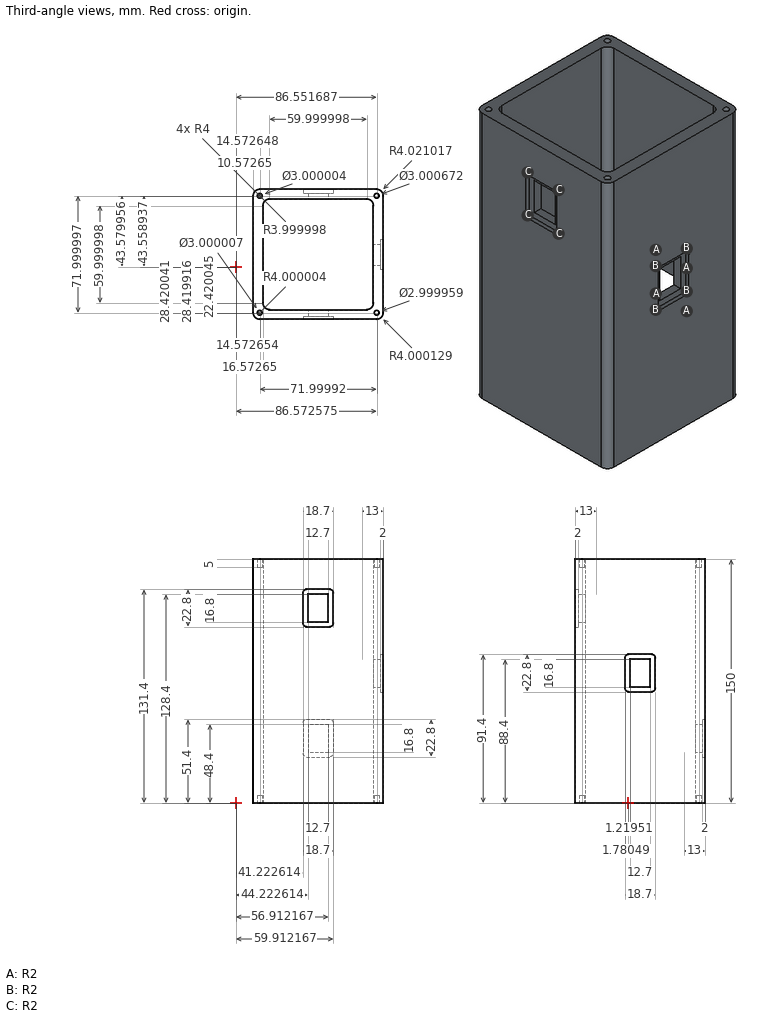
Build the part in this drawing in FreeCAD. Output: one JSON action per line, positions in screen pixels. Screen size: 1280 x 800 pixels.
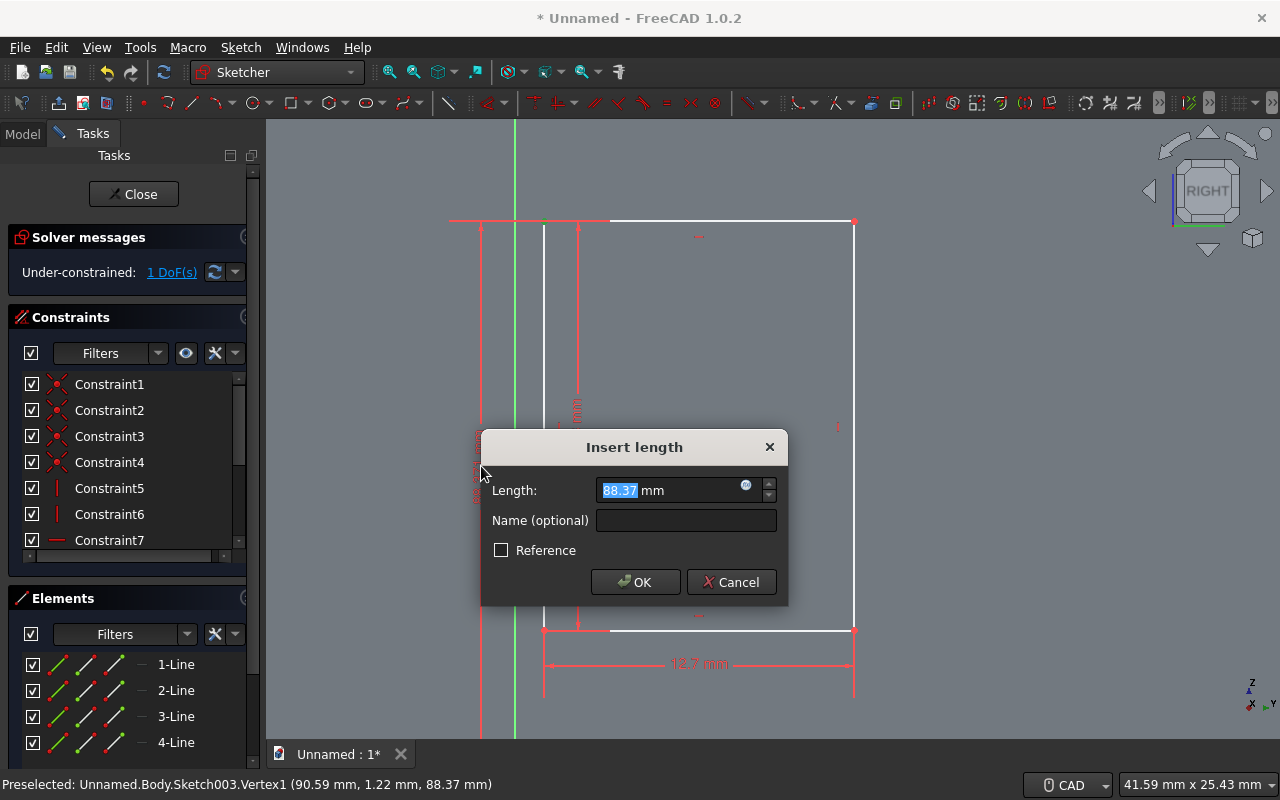
{"action": "type", "text": "88.4"}
{"action": "key", "text": "Return"}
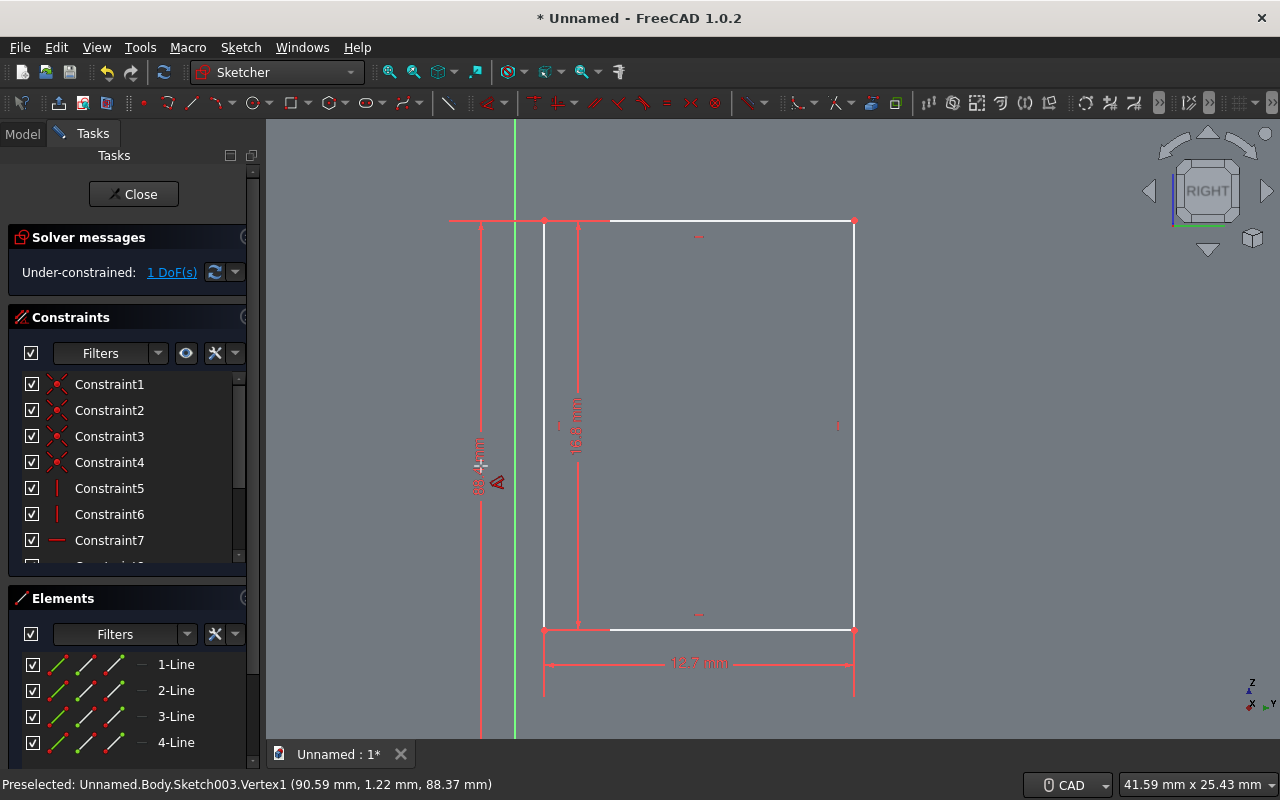
{"action": "scroll", "coordinate": [544, 221], "scroll_direction": "up", "scroll_amount": 2}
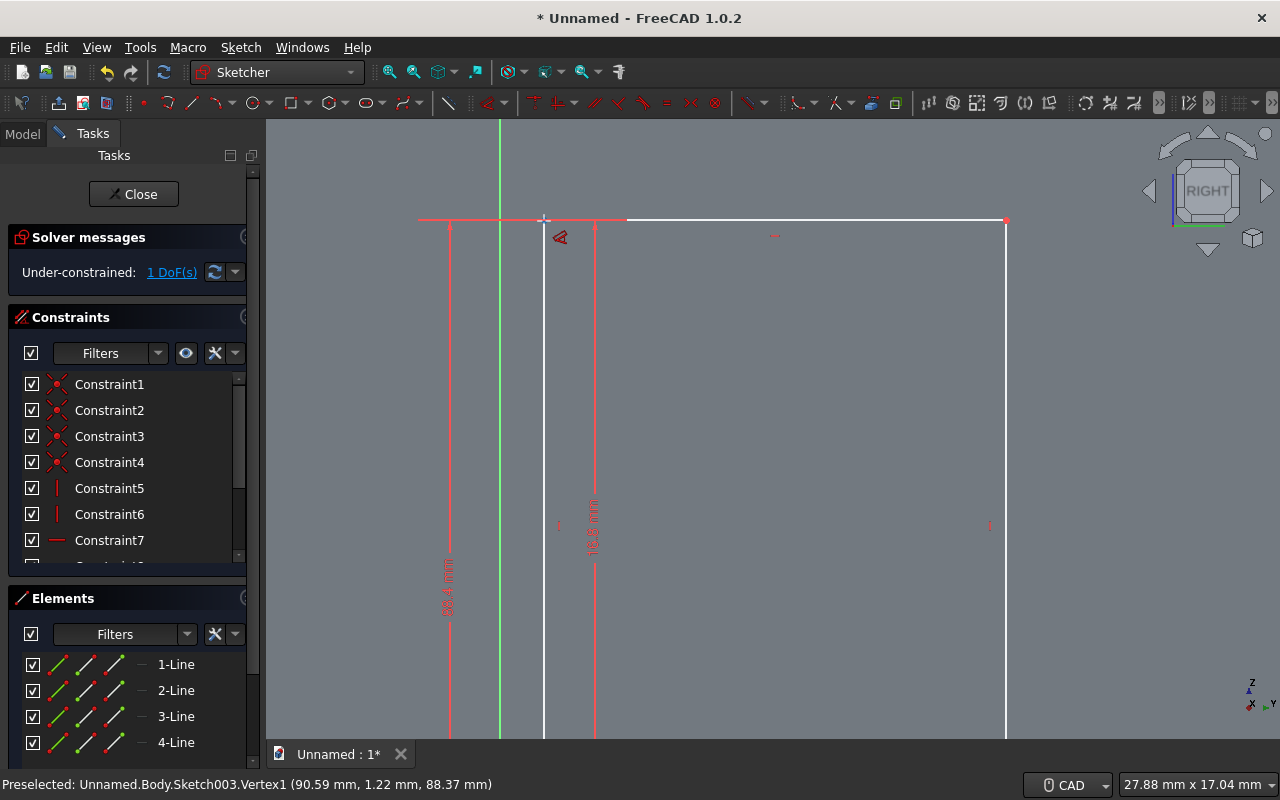
{"action": "left_click", "coordinate": [544, 220]}
{"action": "left_click", "coordinate": [522, 186]}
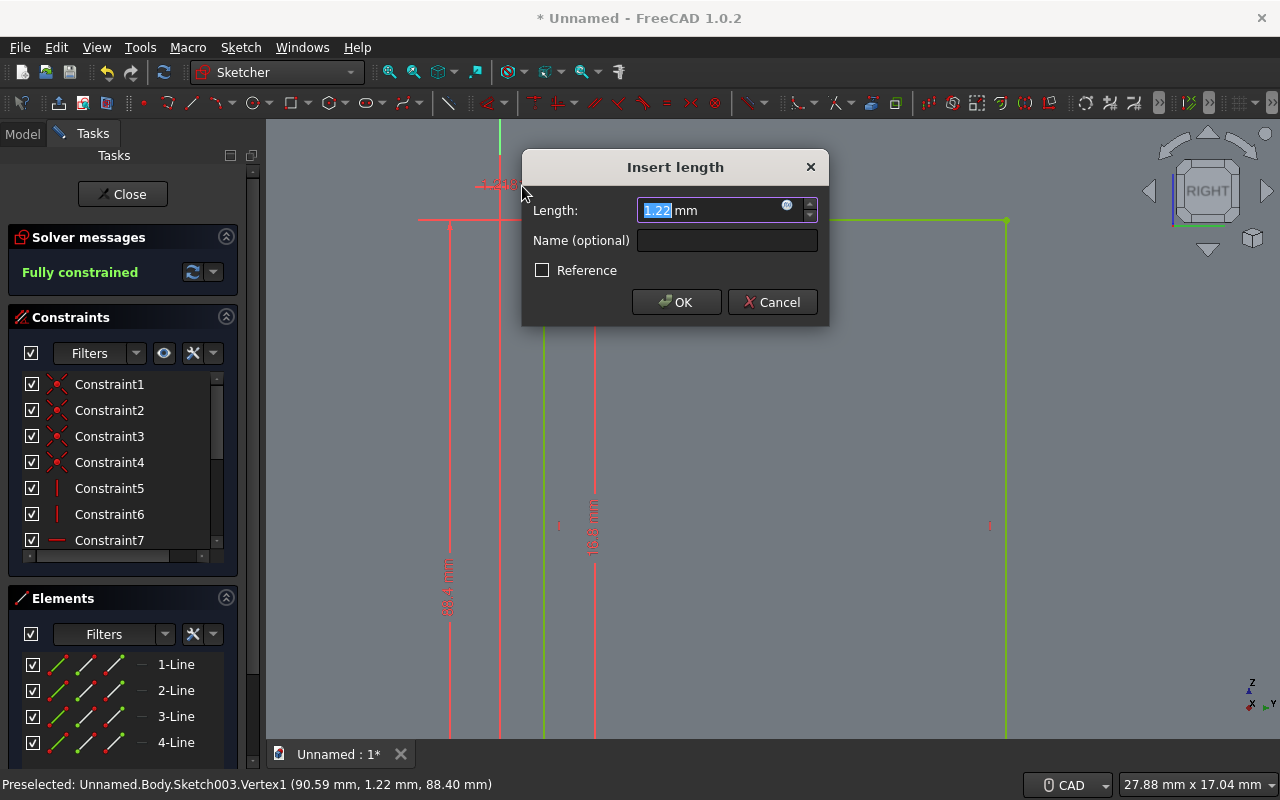
{"action": "type", "text": "1.21951"}
{"action": "key", "text": "Return"}
{"action": "key", "text": "Escape"}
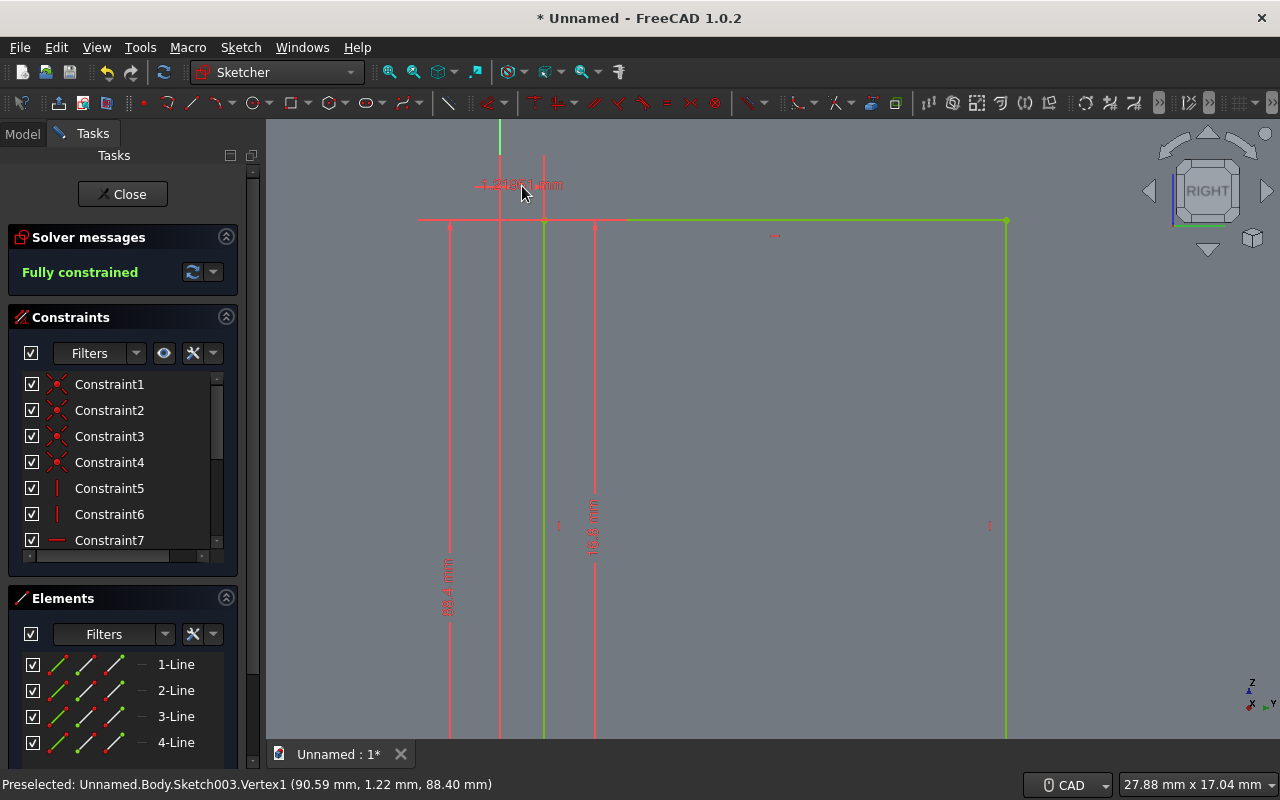
{"action": "left_click", "coordinate": [123, 194]}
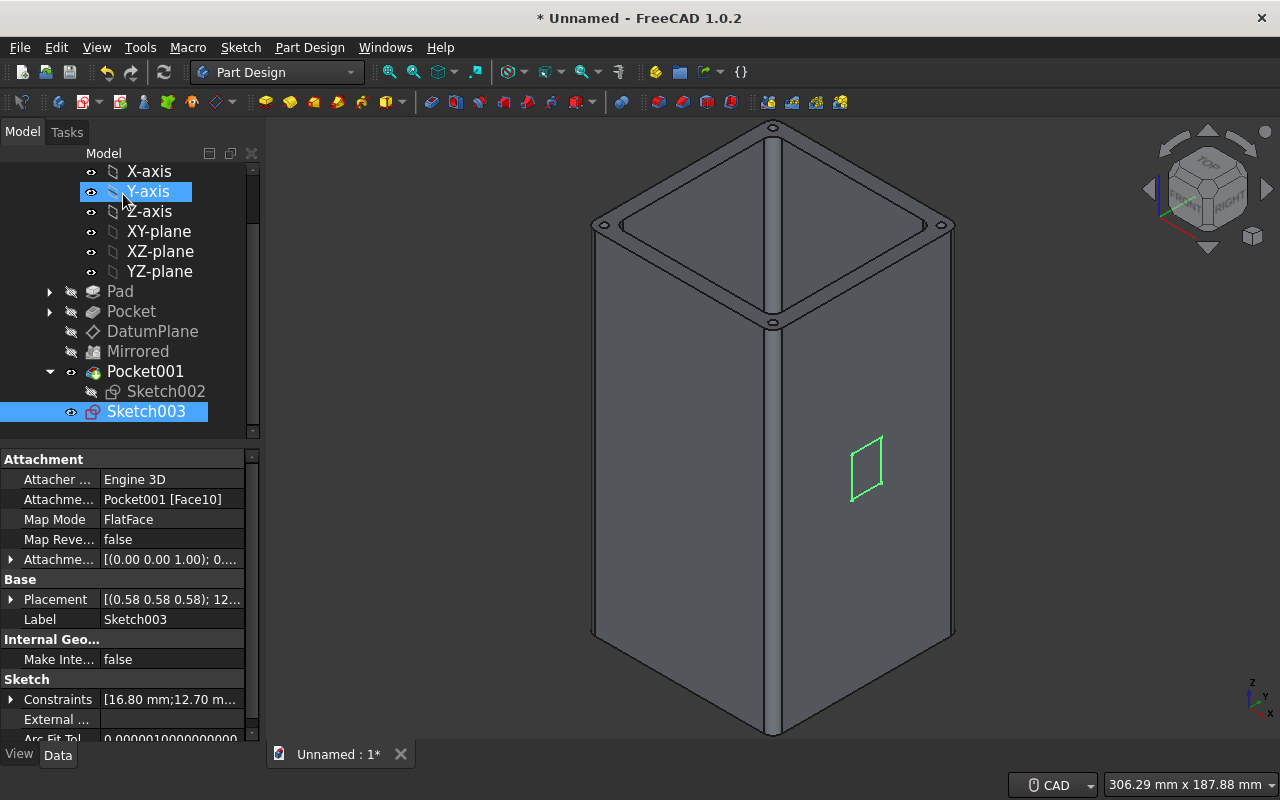
{"action": "left_click", "coordinate": [432, 102]}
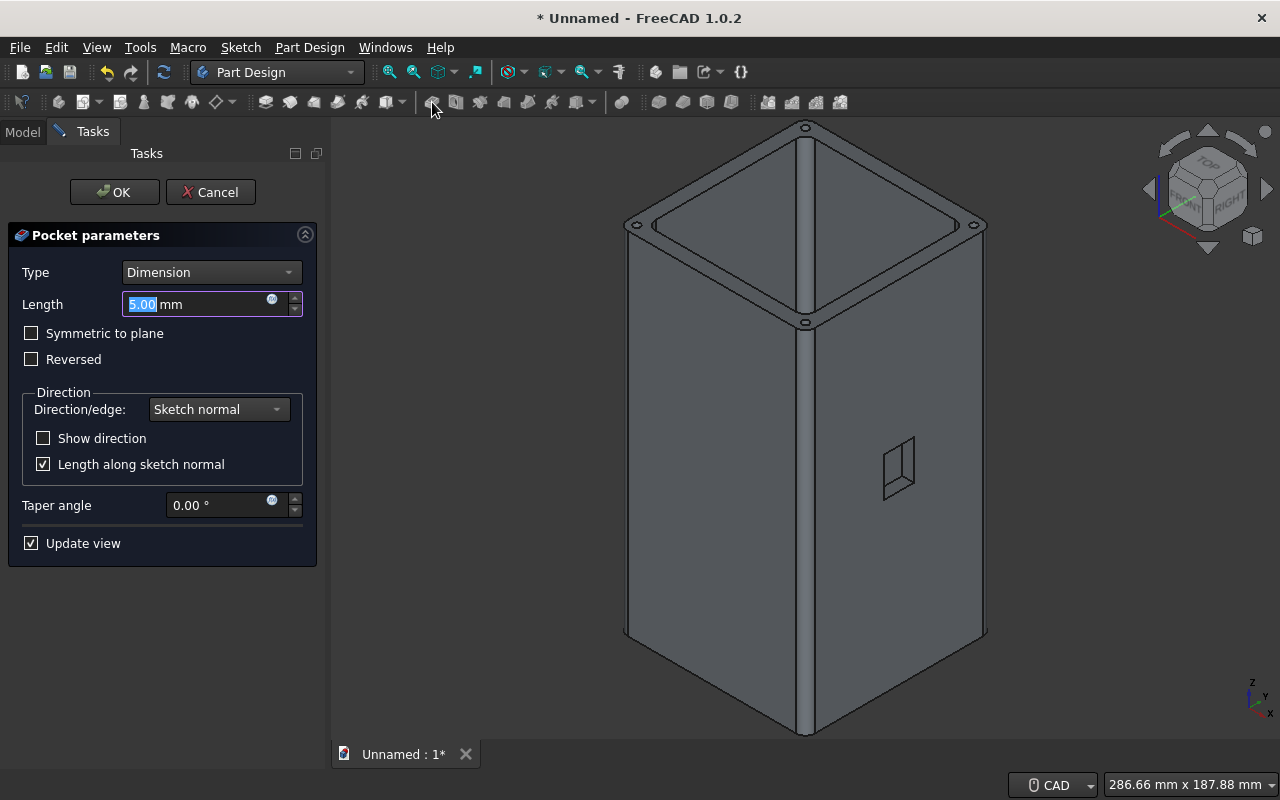
{"action": "type", "text": "13"}
{"action": "key", "text": "Tab"}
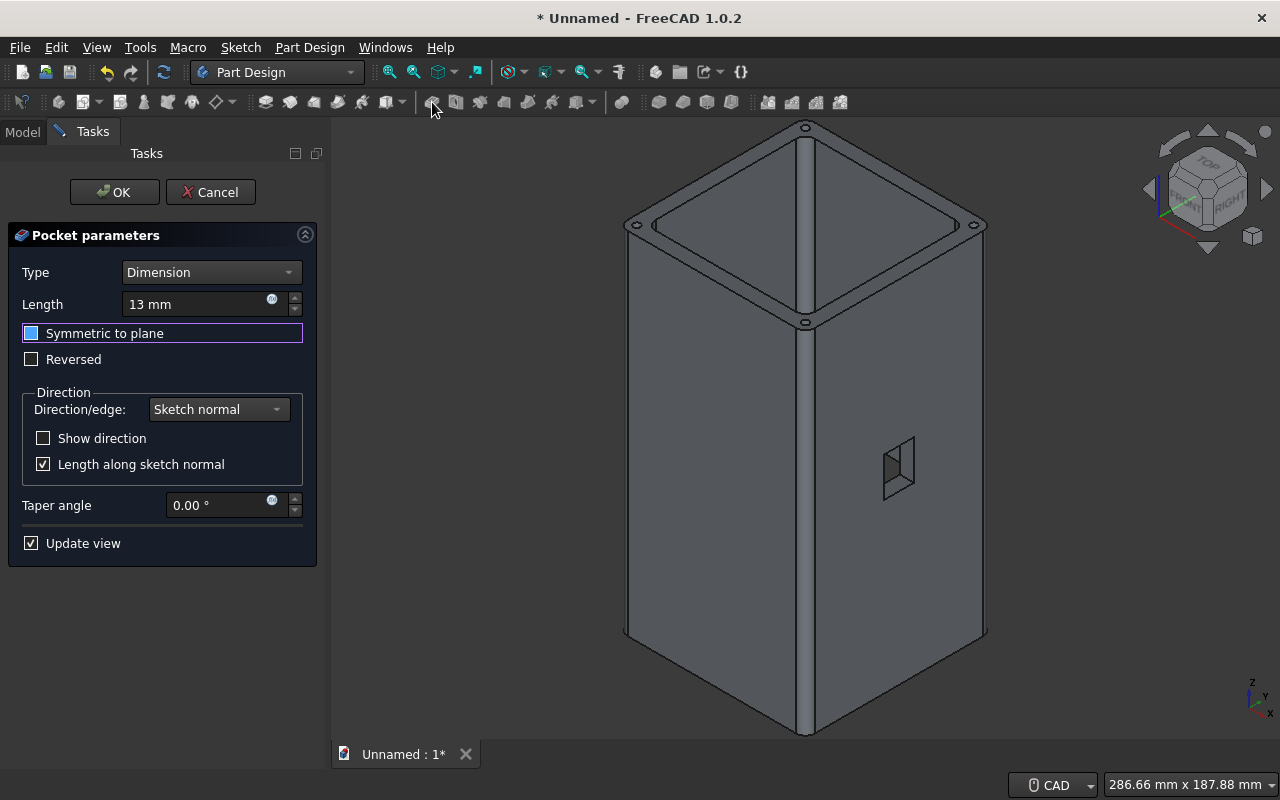
{"action": "left_click", "coordinate": [115, 192]}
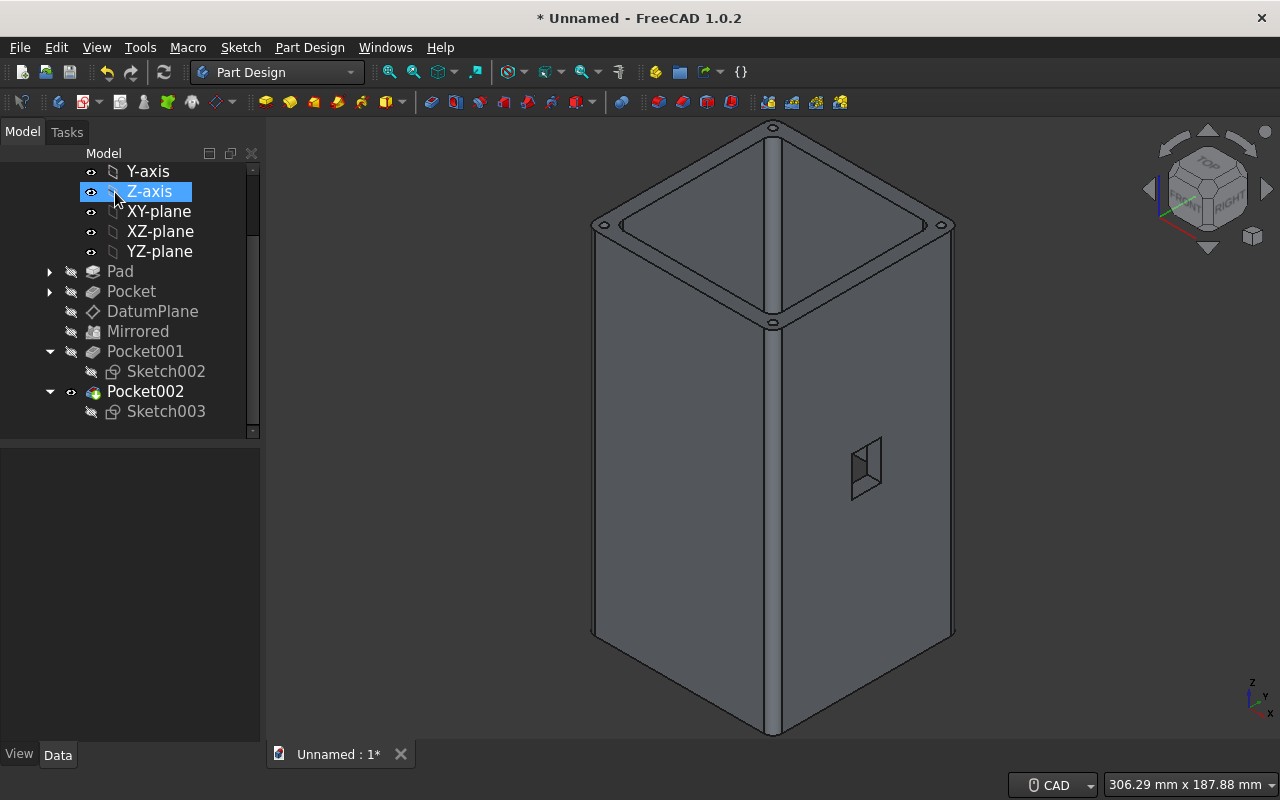
{"action": "left_click", "coordinate": [390, 72]}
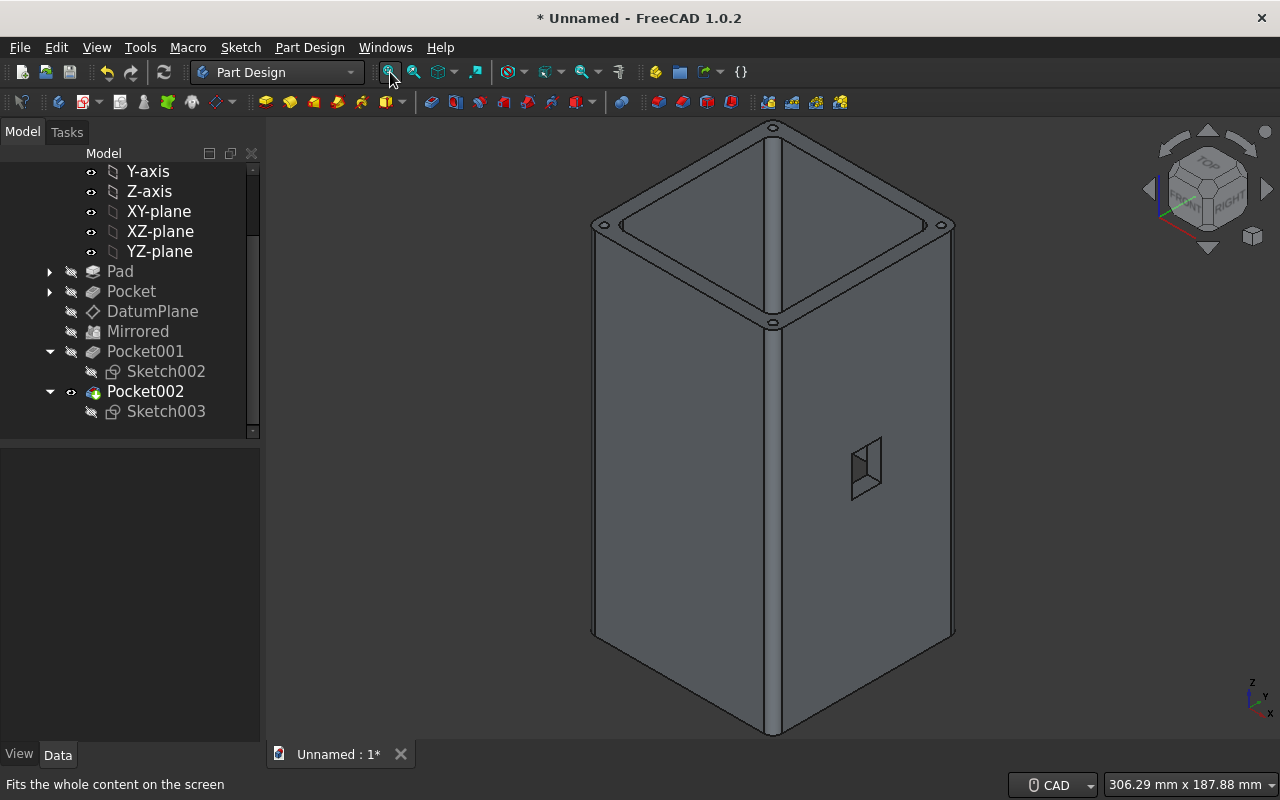
{"action": "left_click", "coordinate": [679, 423]}